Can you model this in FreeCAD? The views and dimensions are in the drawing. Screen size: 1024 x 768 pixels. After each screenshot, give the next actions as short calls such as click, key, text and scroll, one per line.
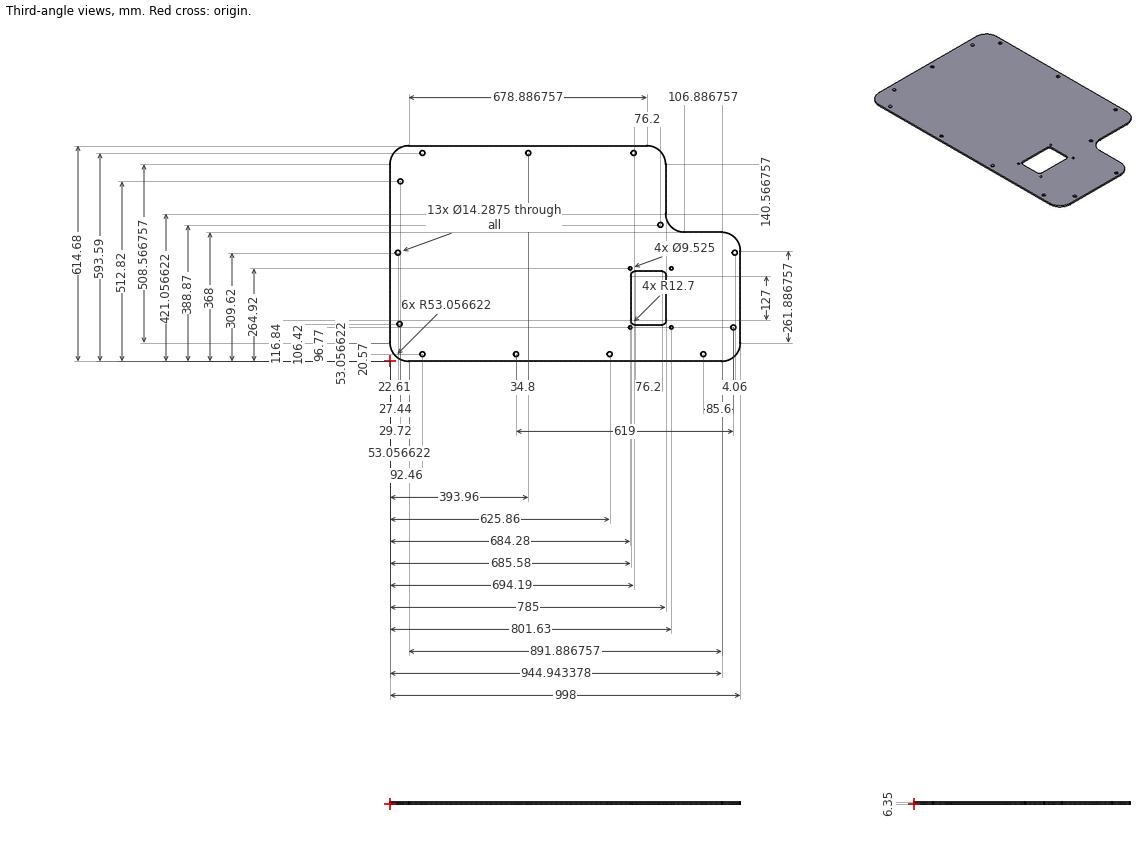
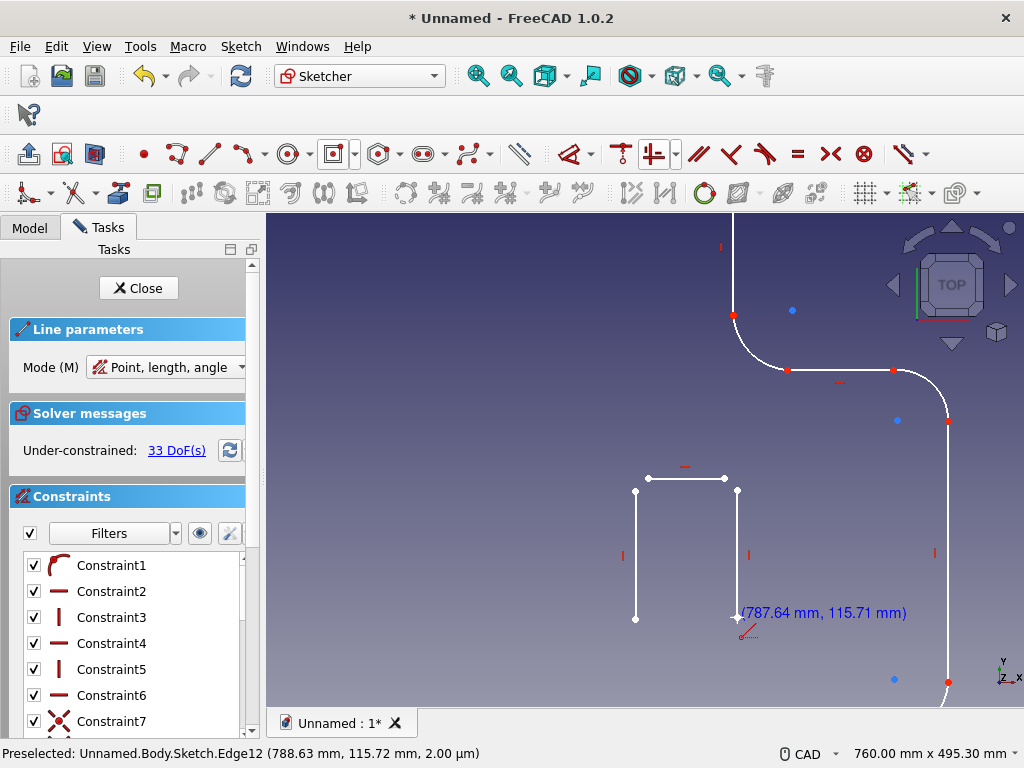
click(724, 630)
click(648, 630)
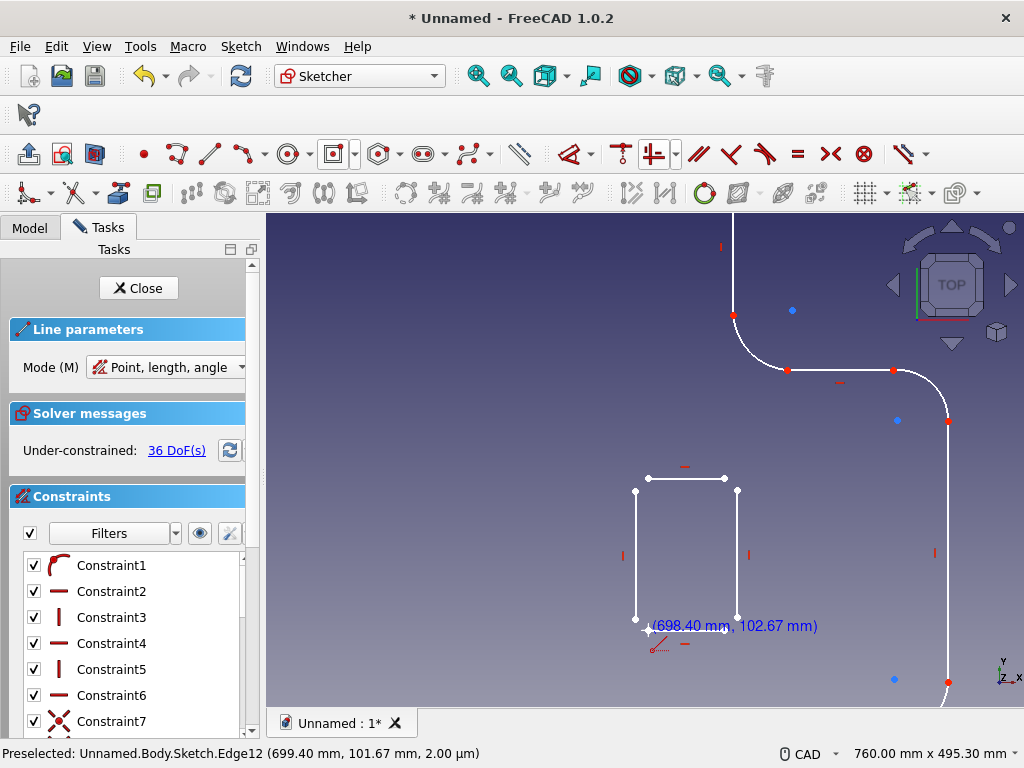
click(242, 154)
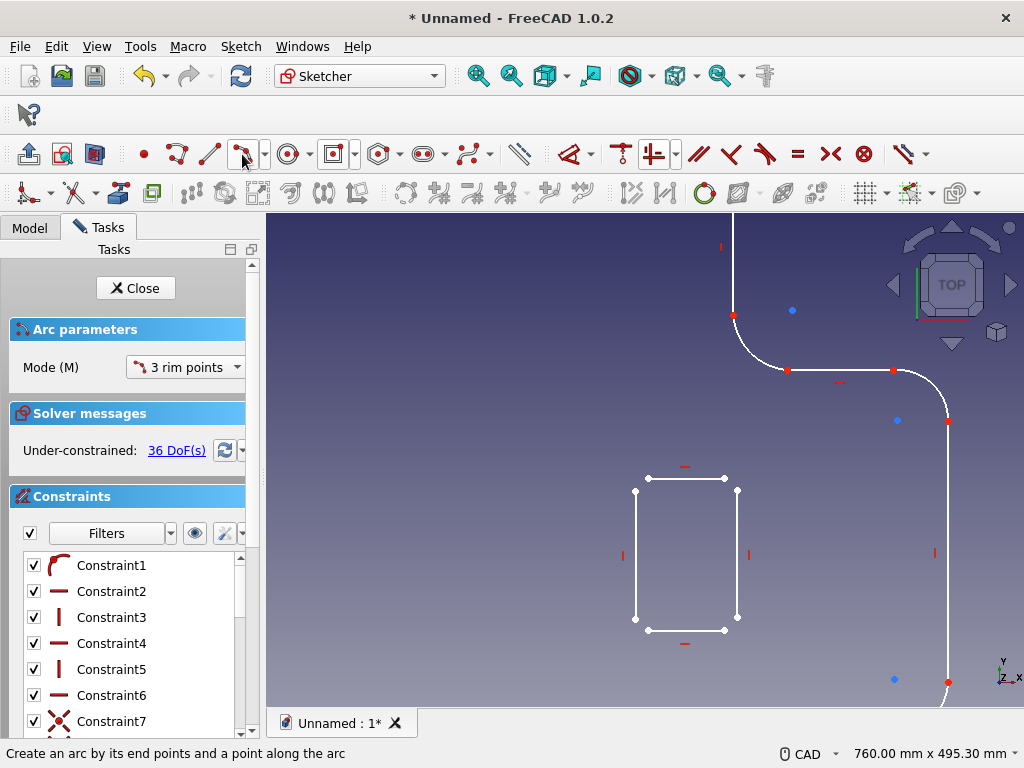
click(636, 492)
click(648, 479)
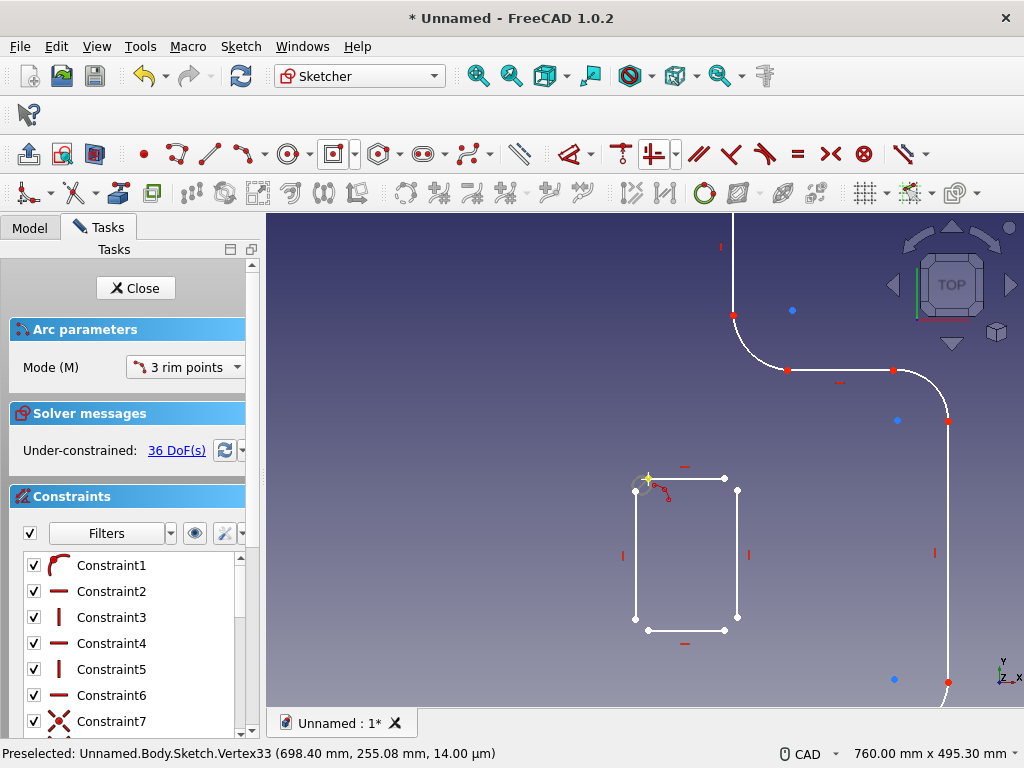
scroll(639, 481, up, 8)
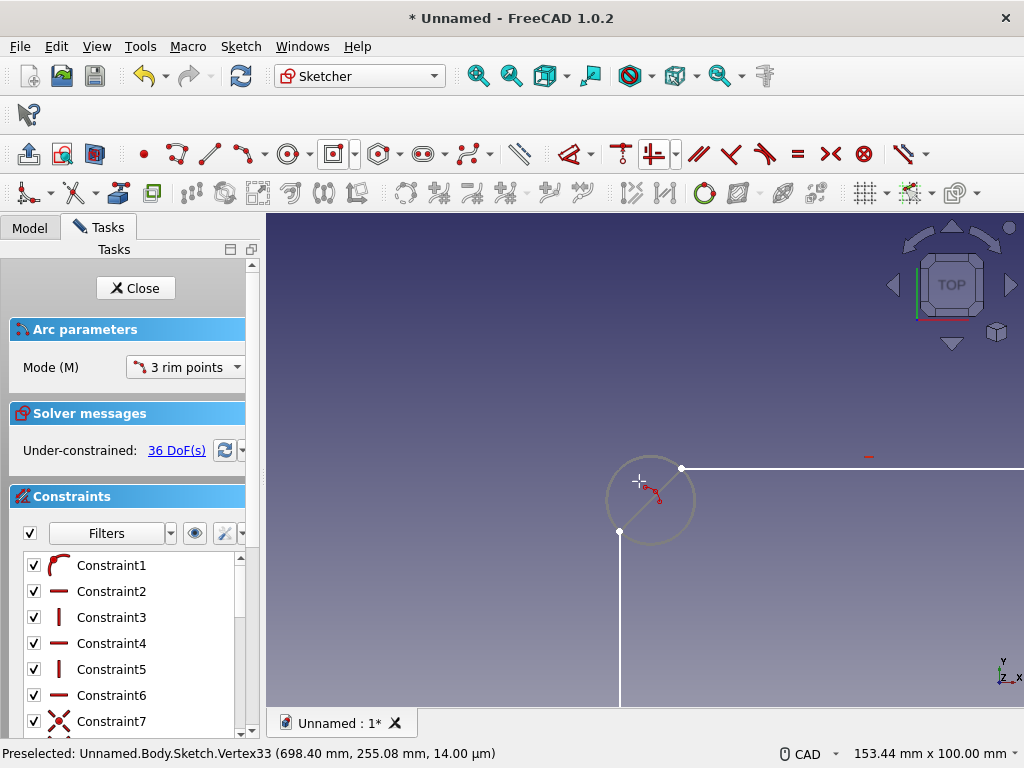
click(637, 480)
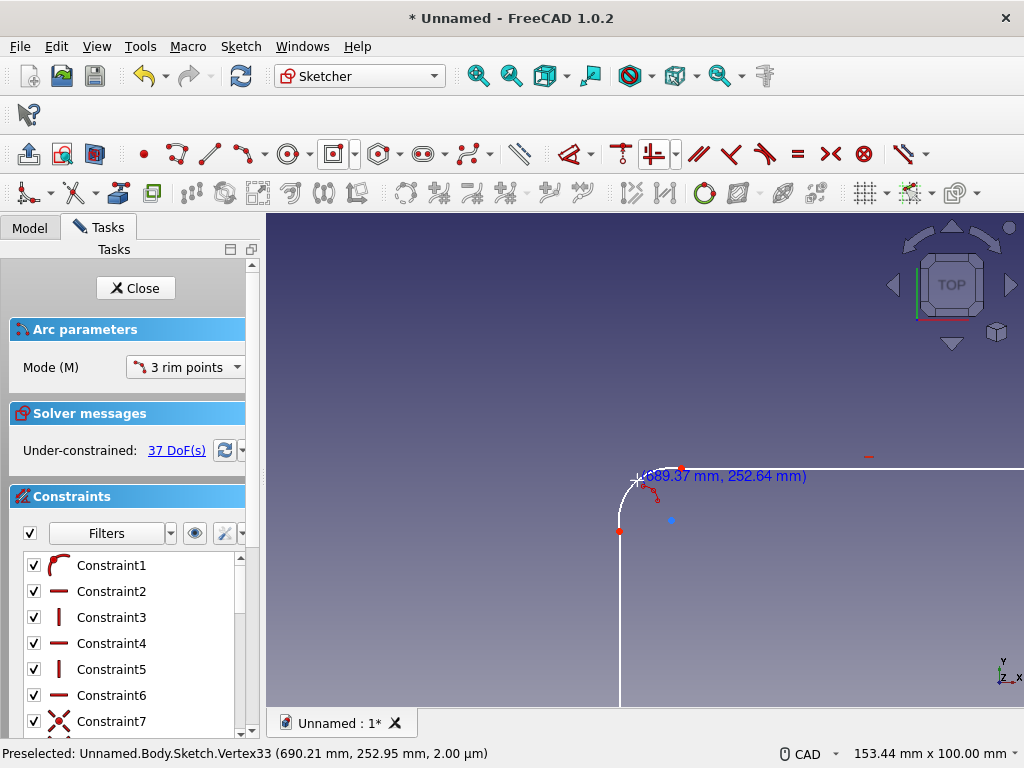
scroll(647, 480, down, 13)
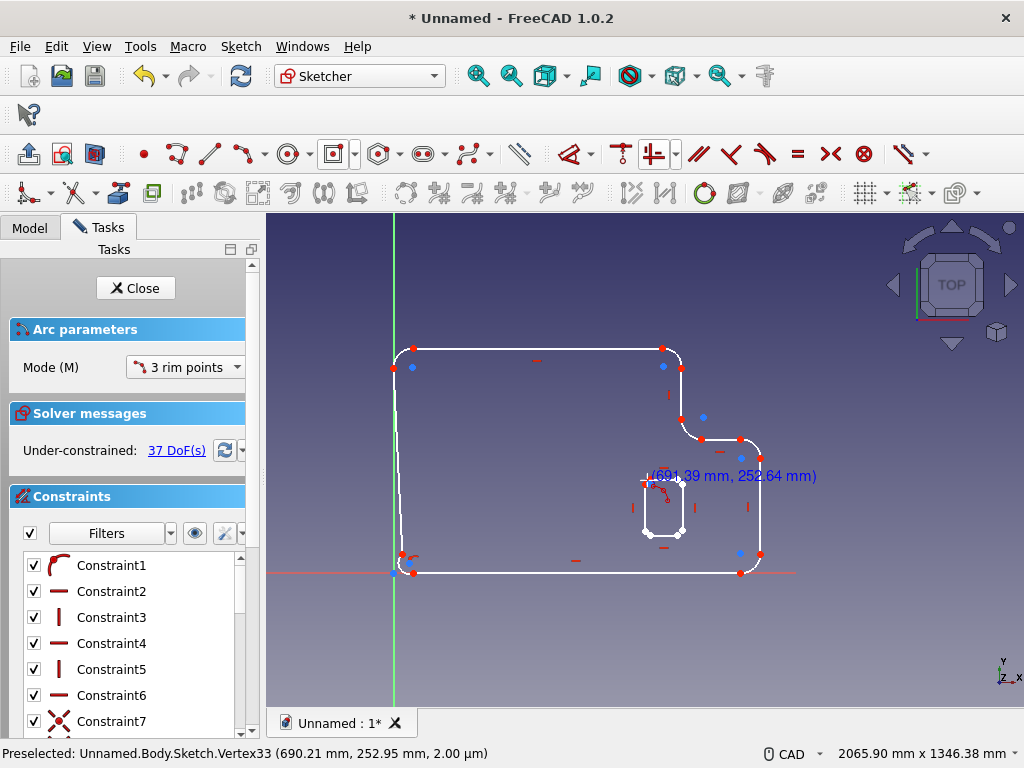
scroll(678, 479, up, 5)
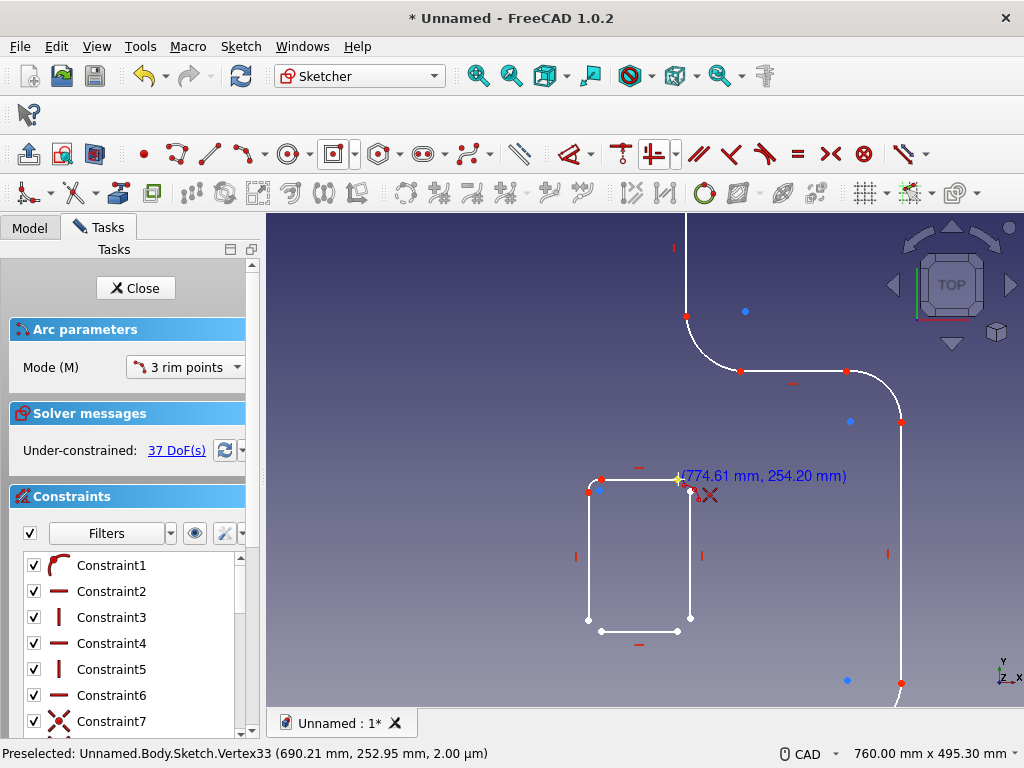
click(677, 480)
click(690, 492)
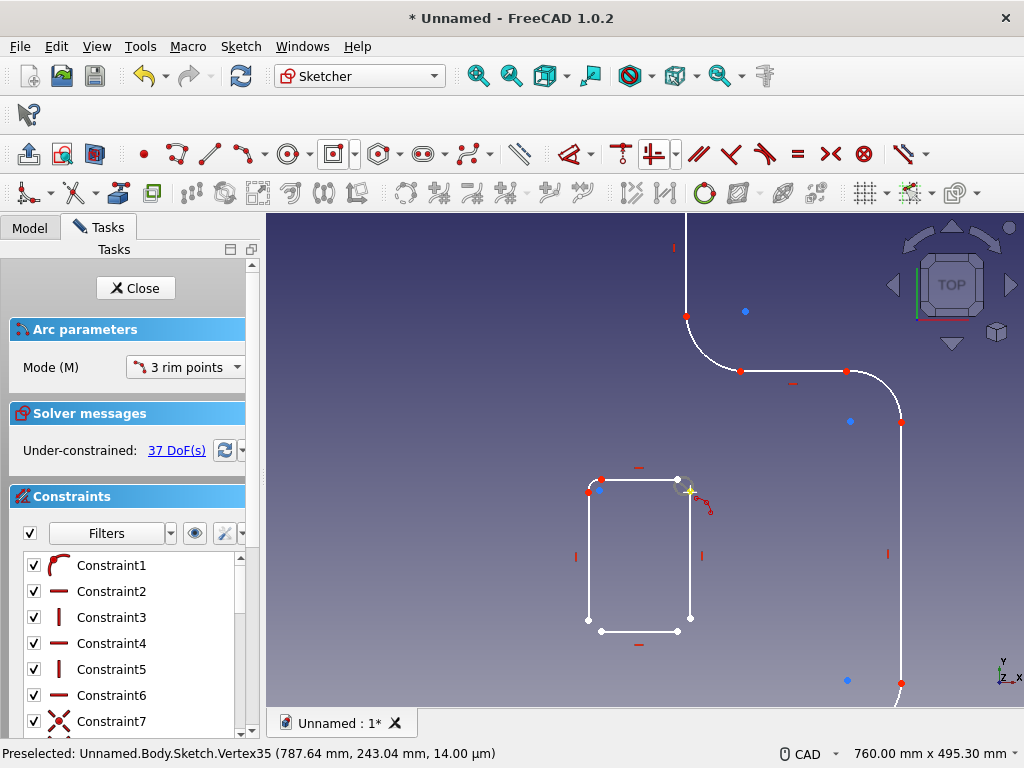
scroll(686, 482, up, 8)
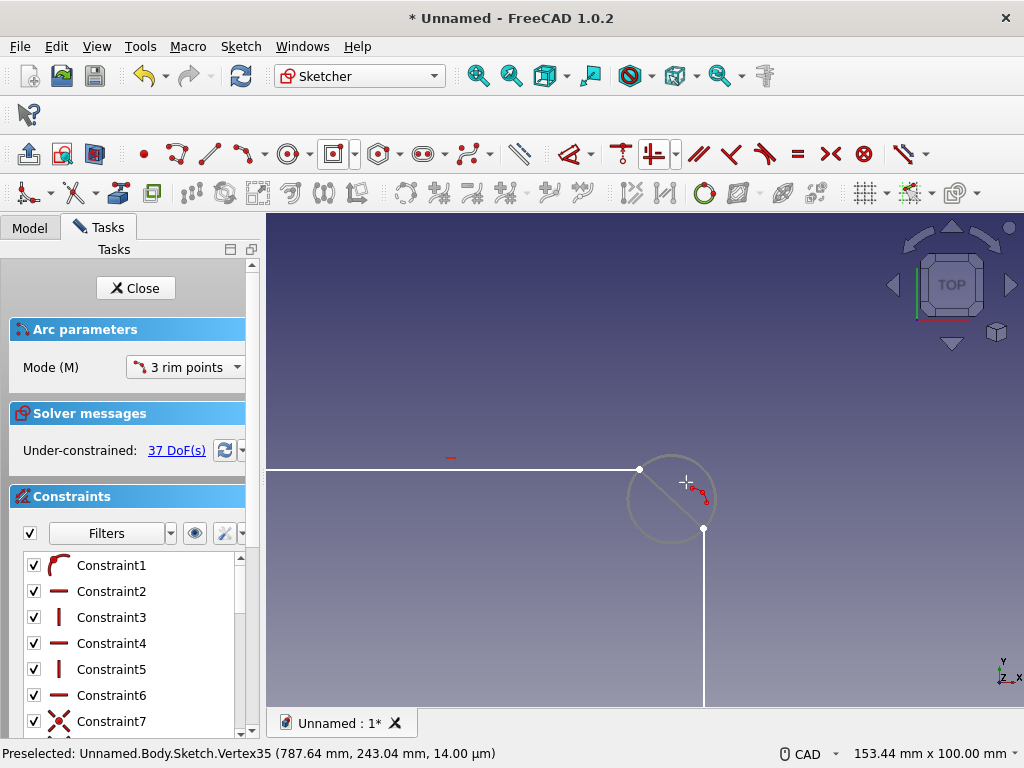
click(683, 481)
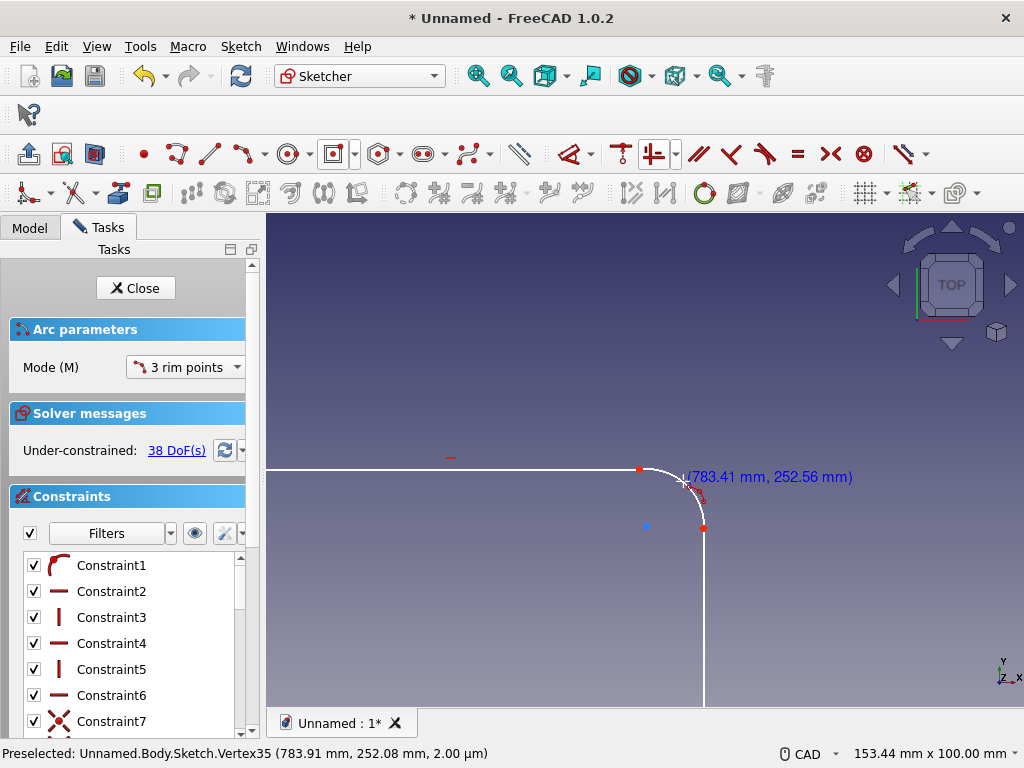
scroll(681, 480, down, 13)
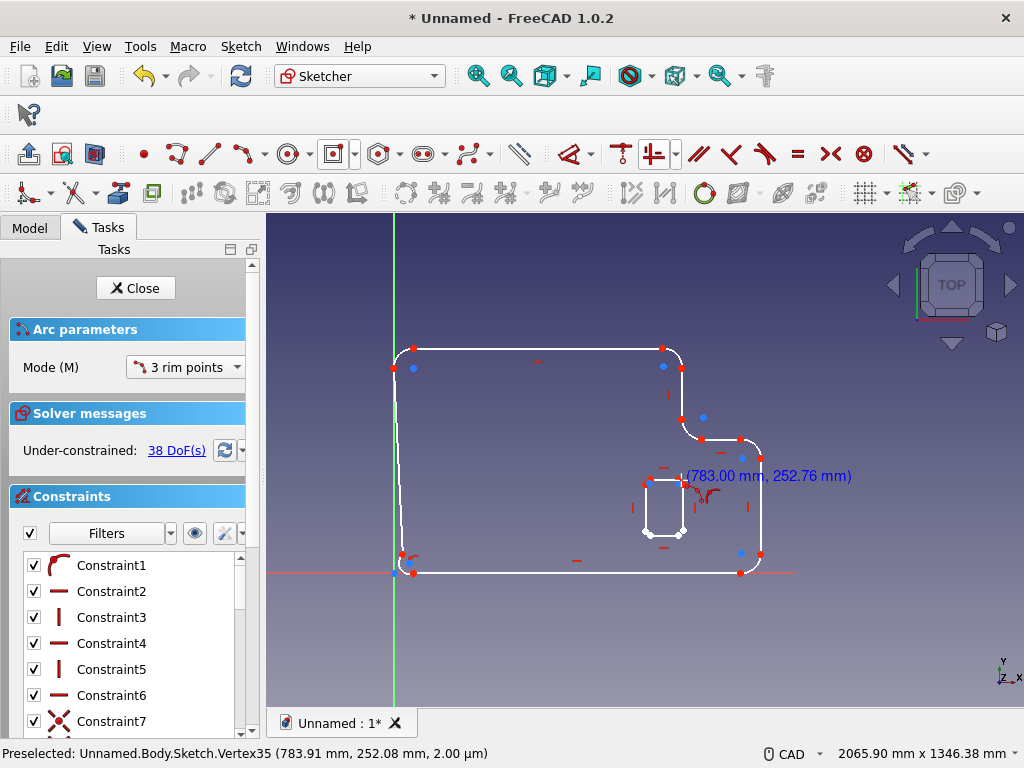
scroll(683, 530, up, 5)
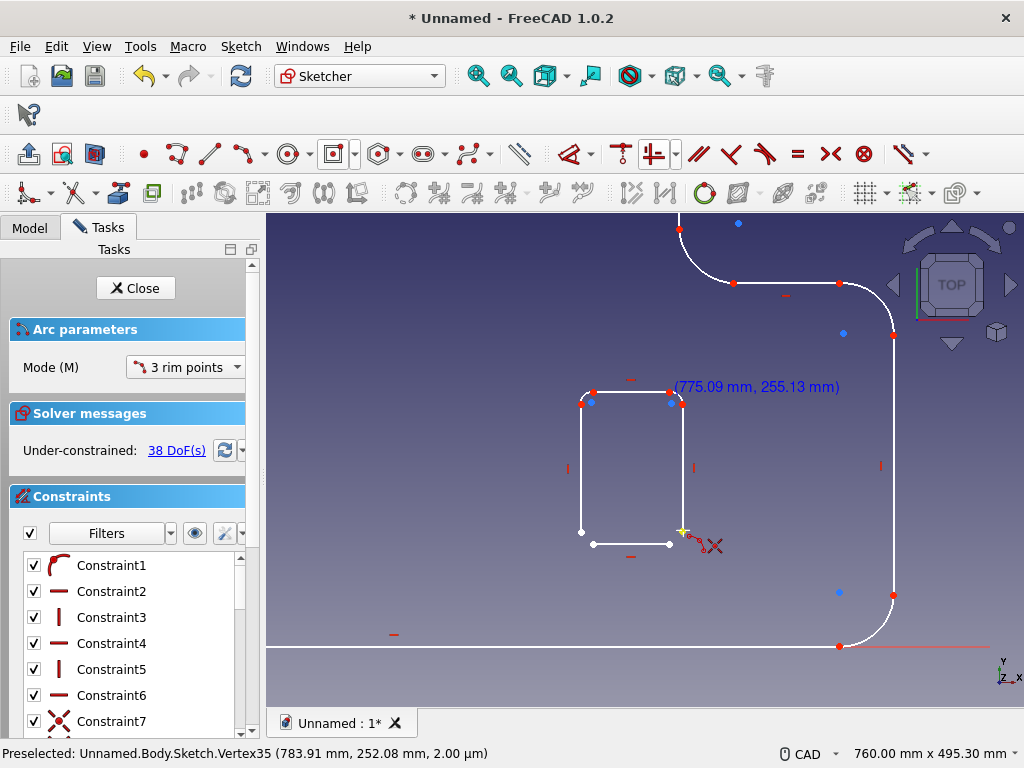
click(683, 531)
click(670, 544)